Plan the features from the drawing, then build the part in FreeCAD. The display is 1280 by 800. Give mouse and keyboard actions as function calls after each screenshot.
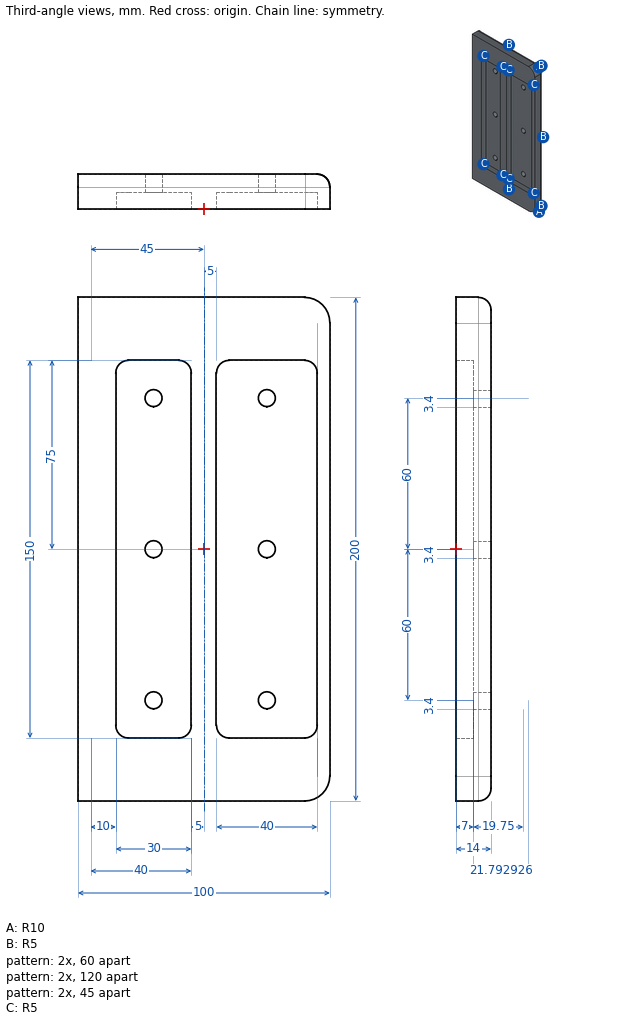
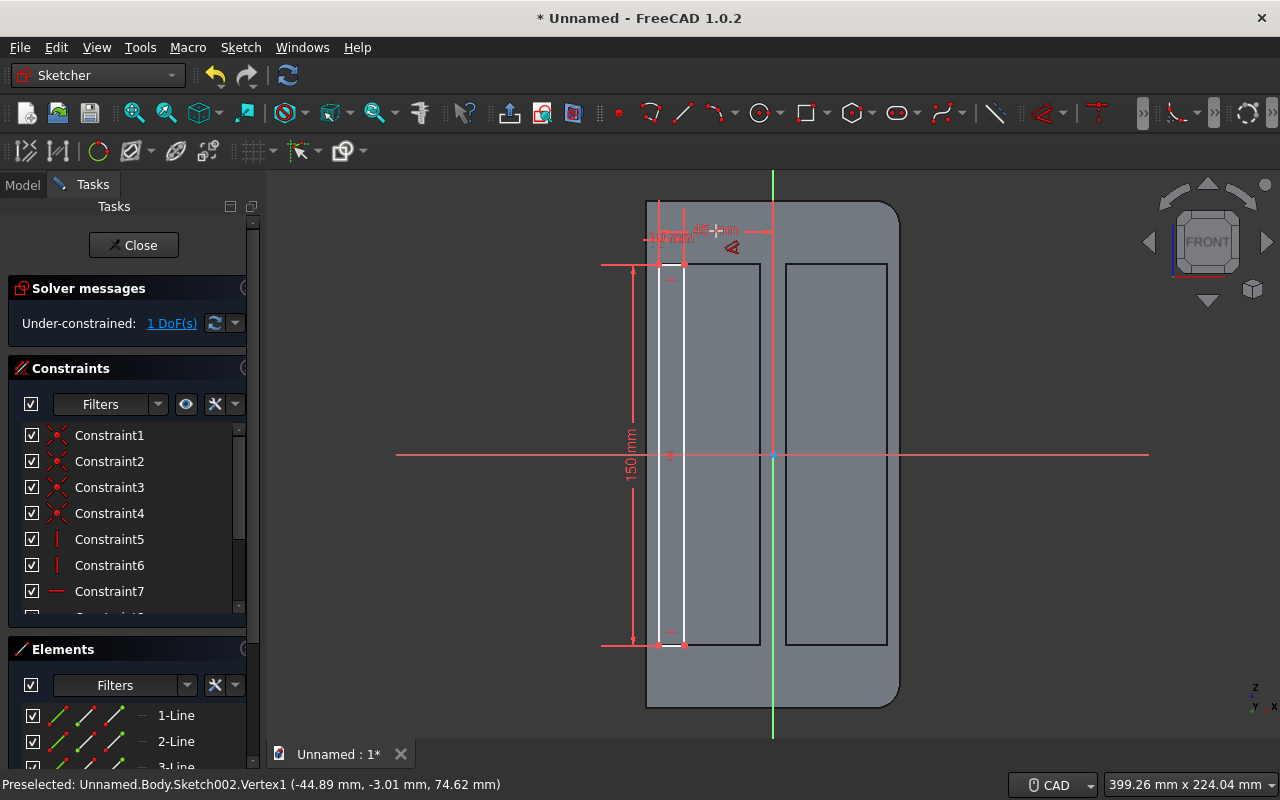
click(659, 265)
click(807, 360)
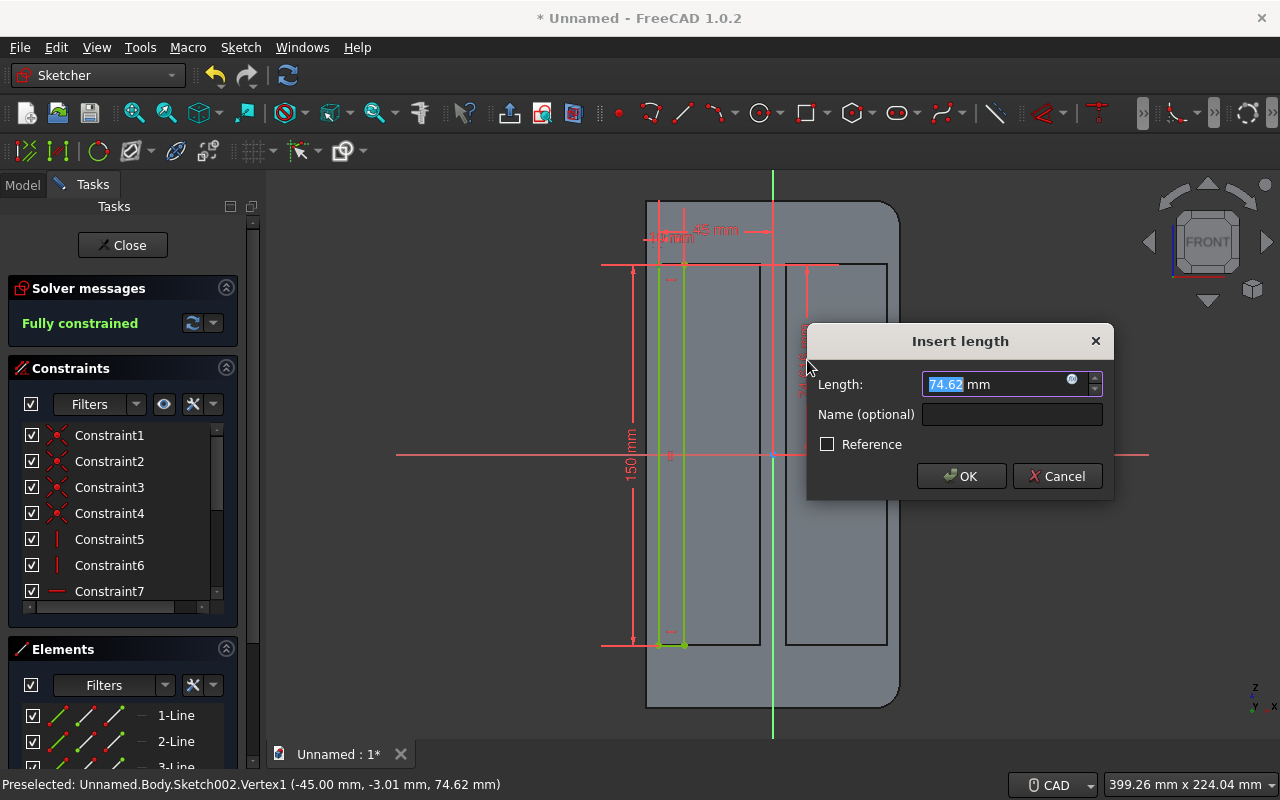
text(75)
key(Return)
key(Escape)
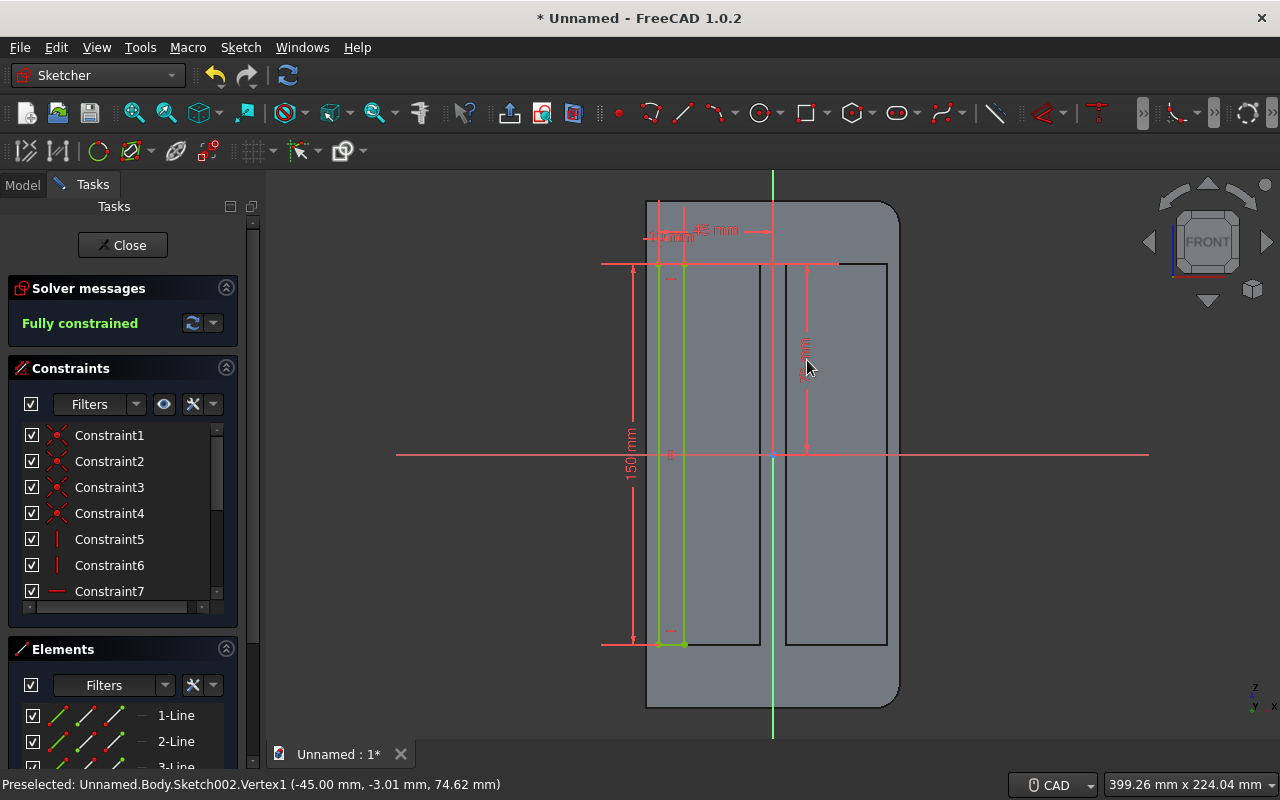
click(123, 245)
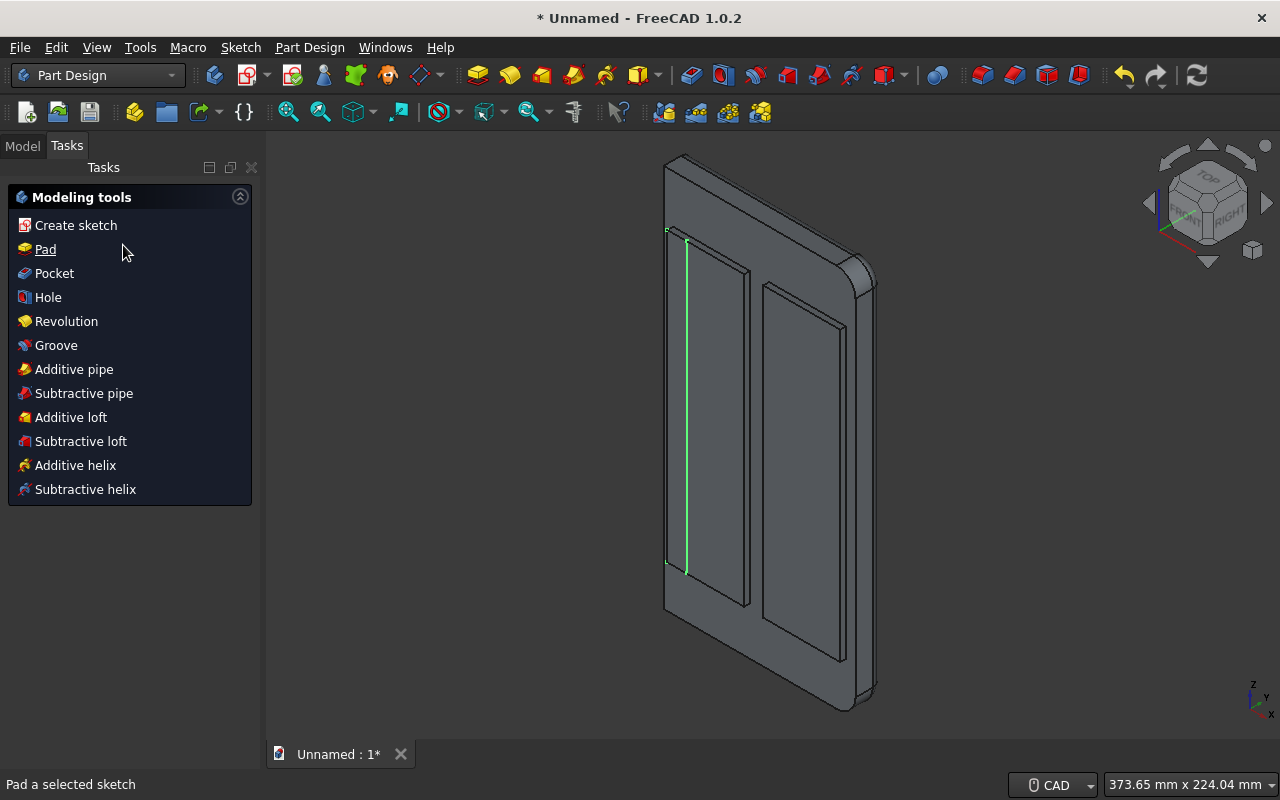
click(692, 76)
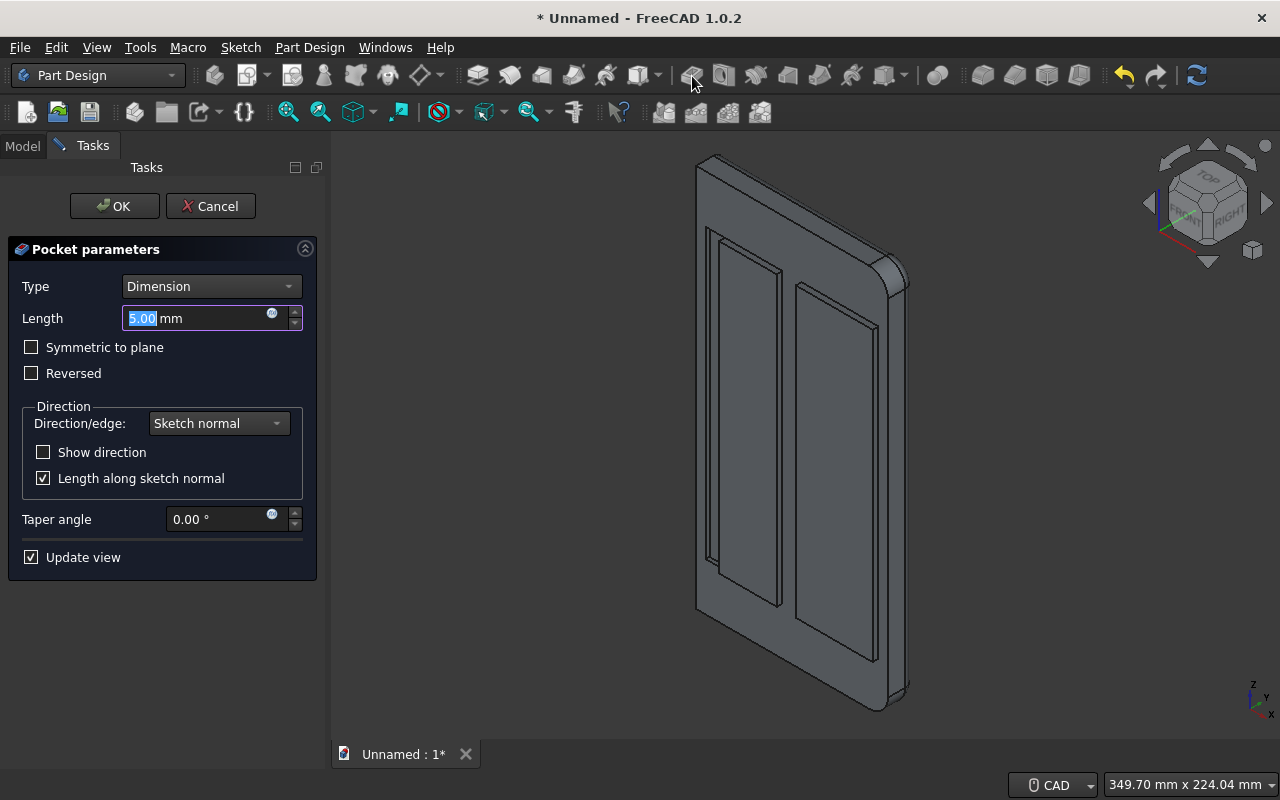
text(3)
key(Tab)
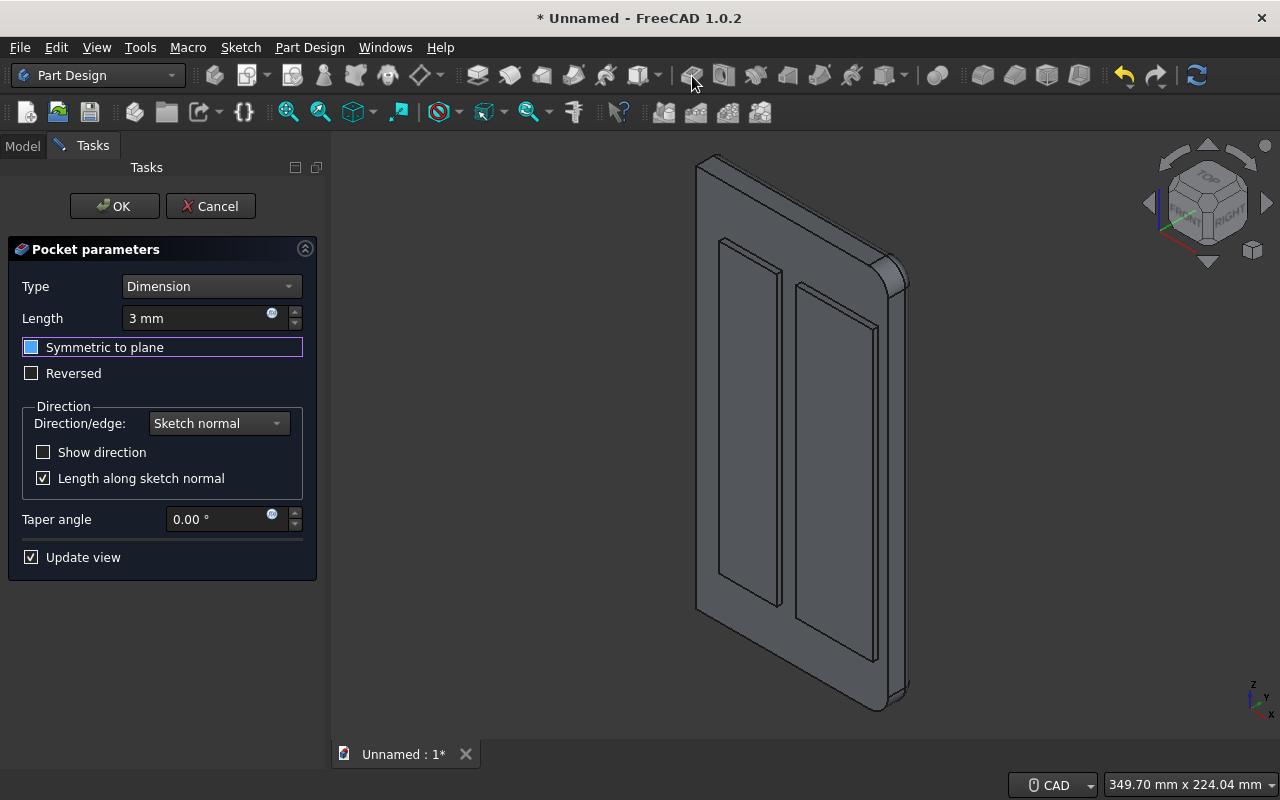
click(115, 206)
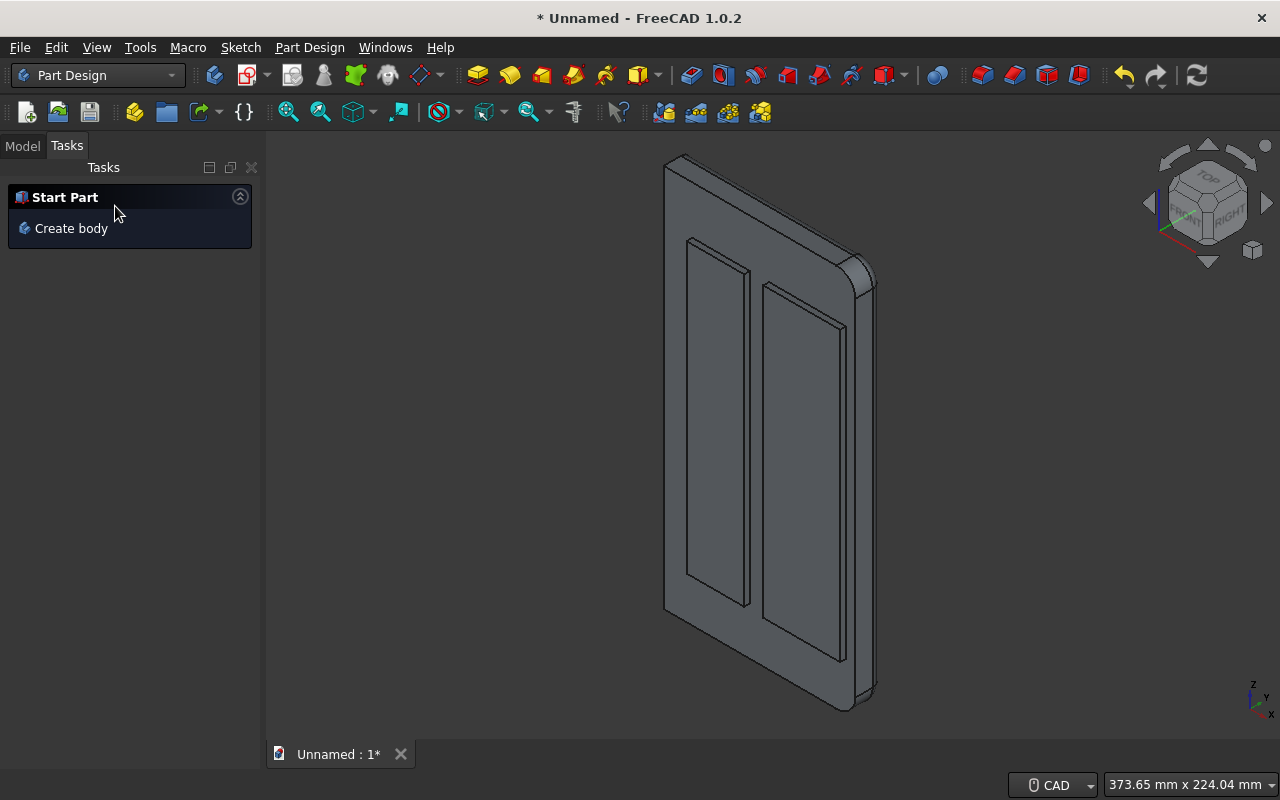
click(802, 378)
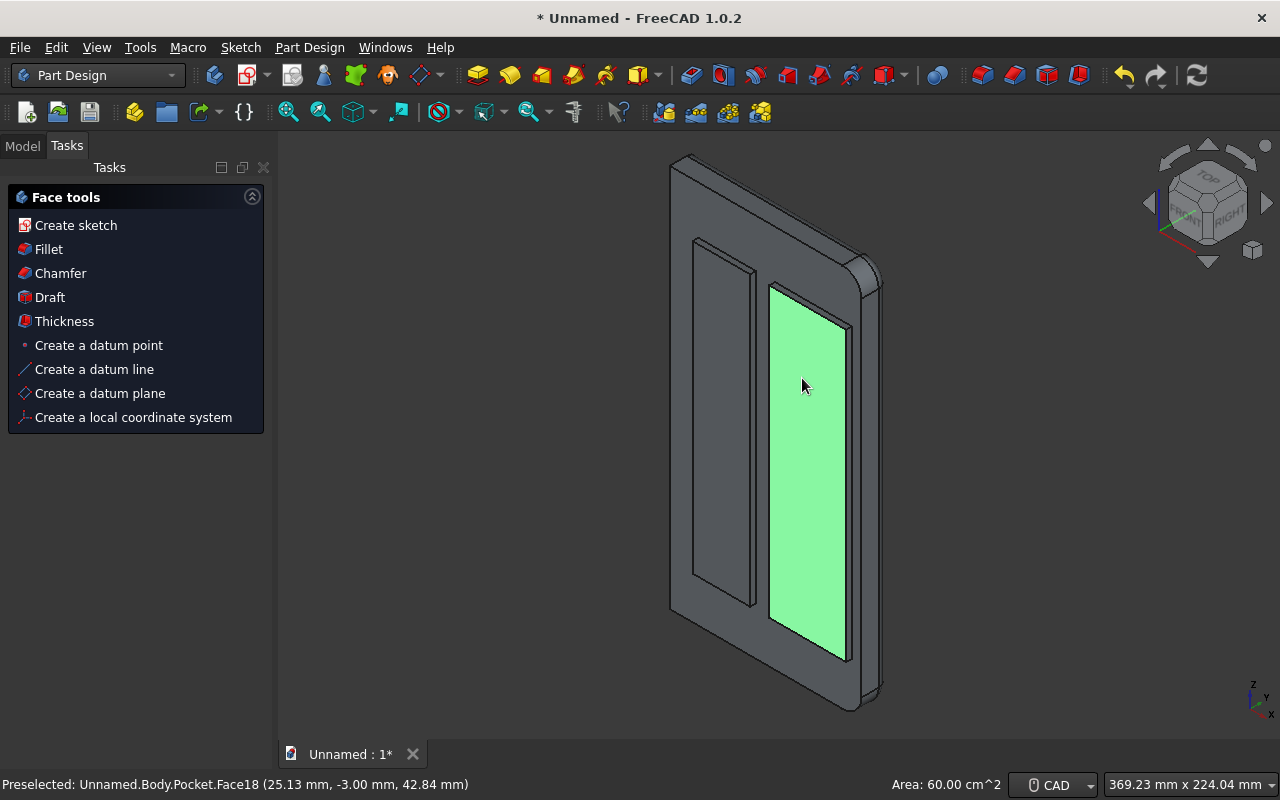
click(248, 76)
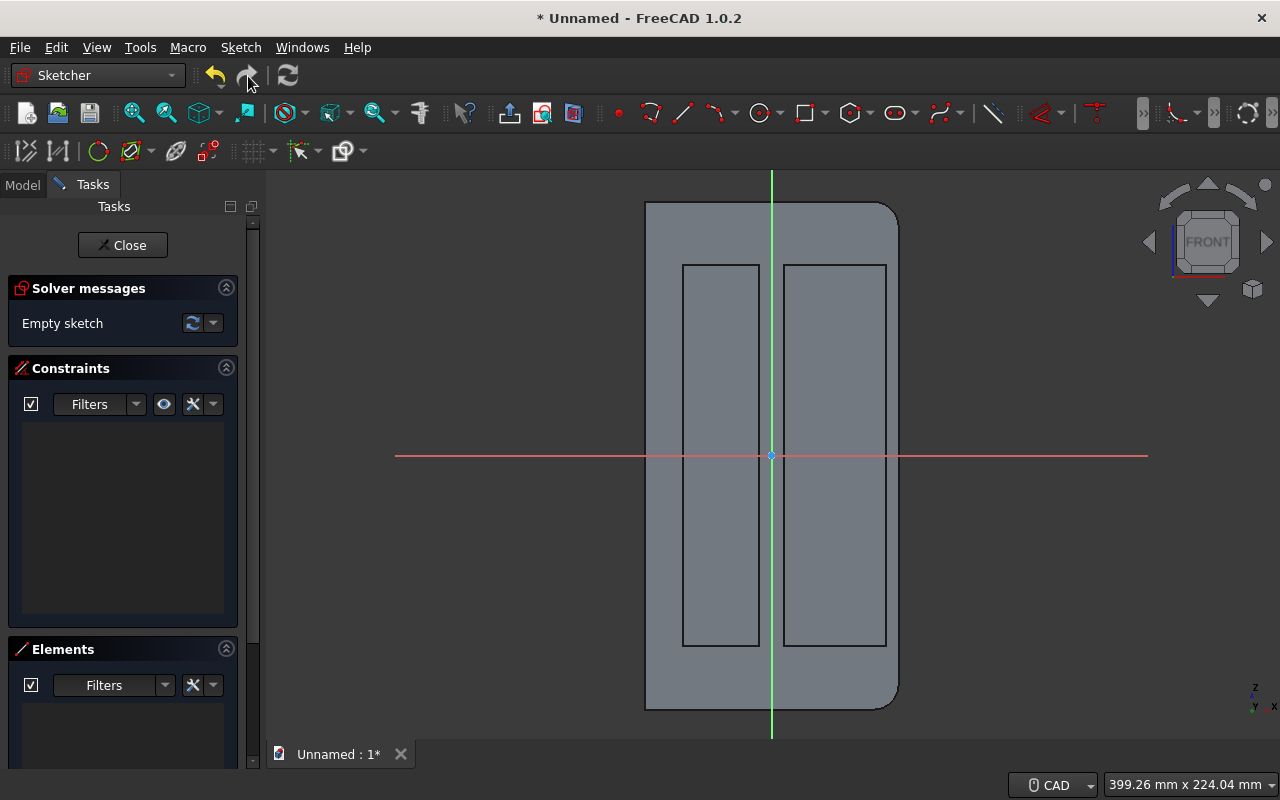
click(806, 114)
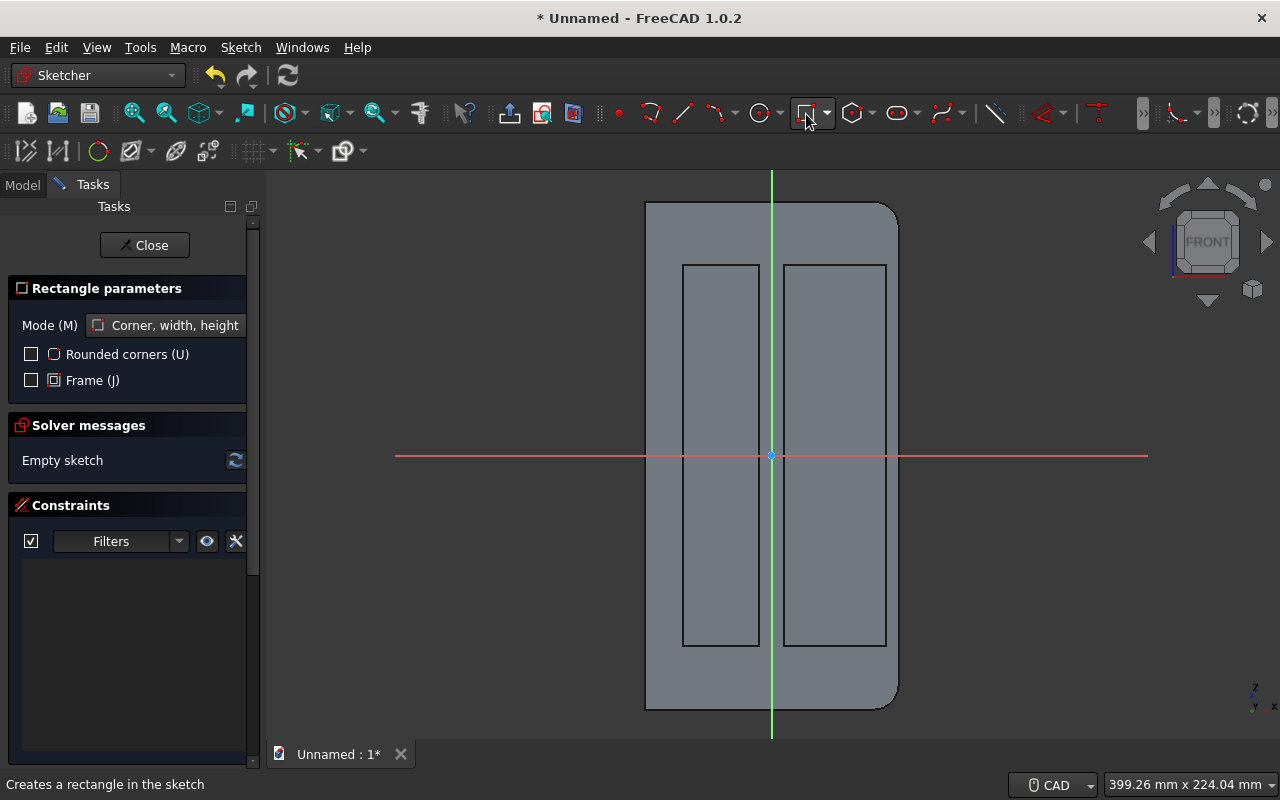
scroll(784, 265, up, 2)